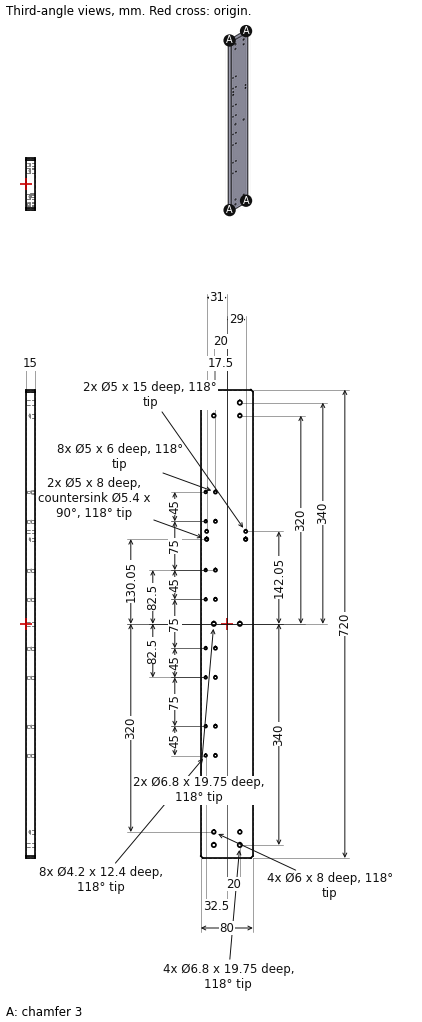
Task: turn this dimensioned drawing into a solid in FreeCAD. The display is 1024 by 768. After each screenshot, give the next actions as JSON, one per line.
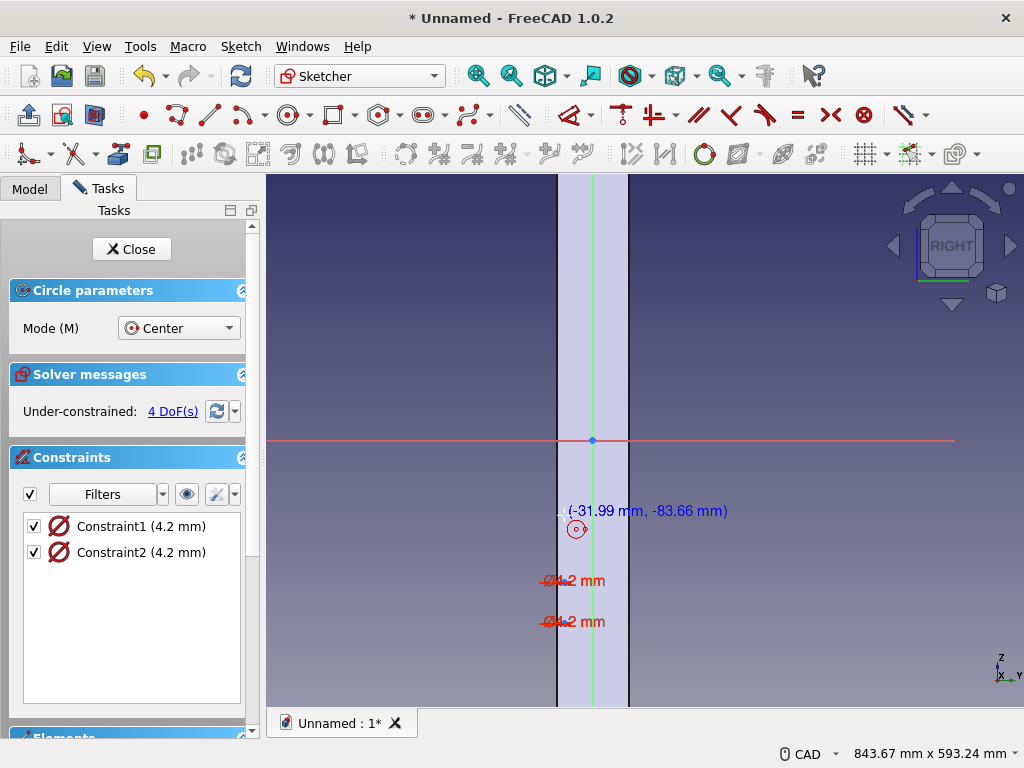
{"action": "left_click", "coordinate": [564, 515]}
{"action": "mouse_move", "coordinate": [565, 514]}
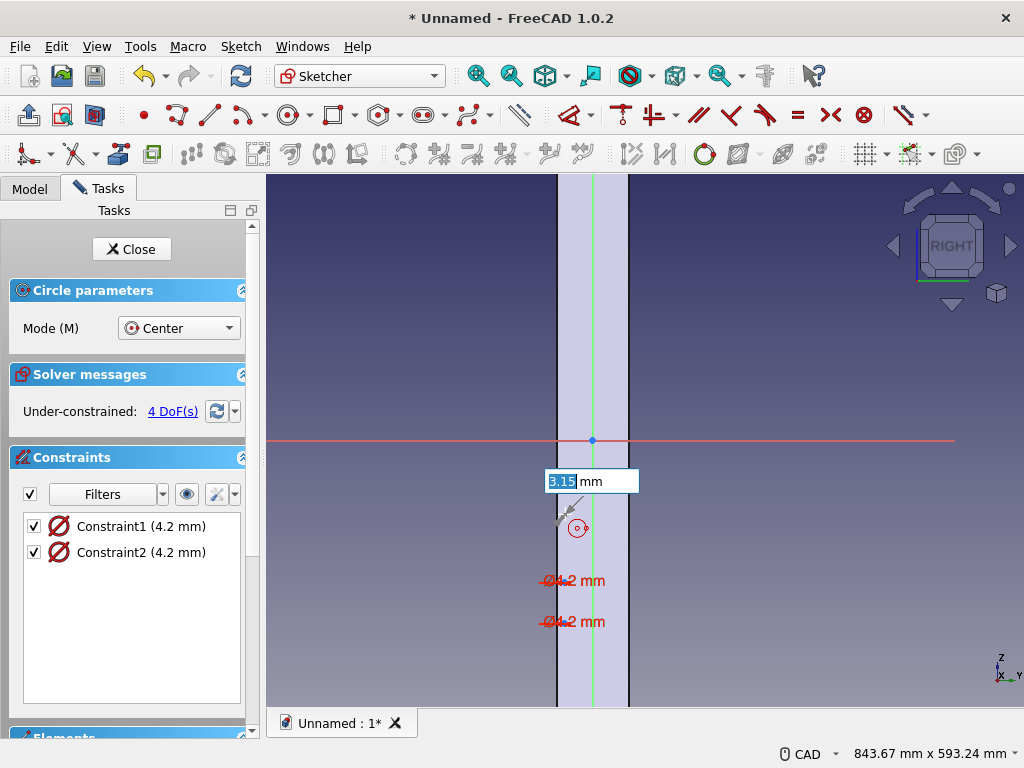
{"action": "type", "text": "4.2"}
{"action": "key", "text": "Return"}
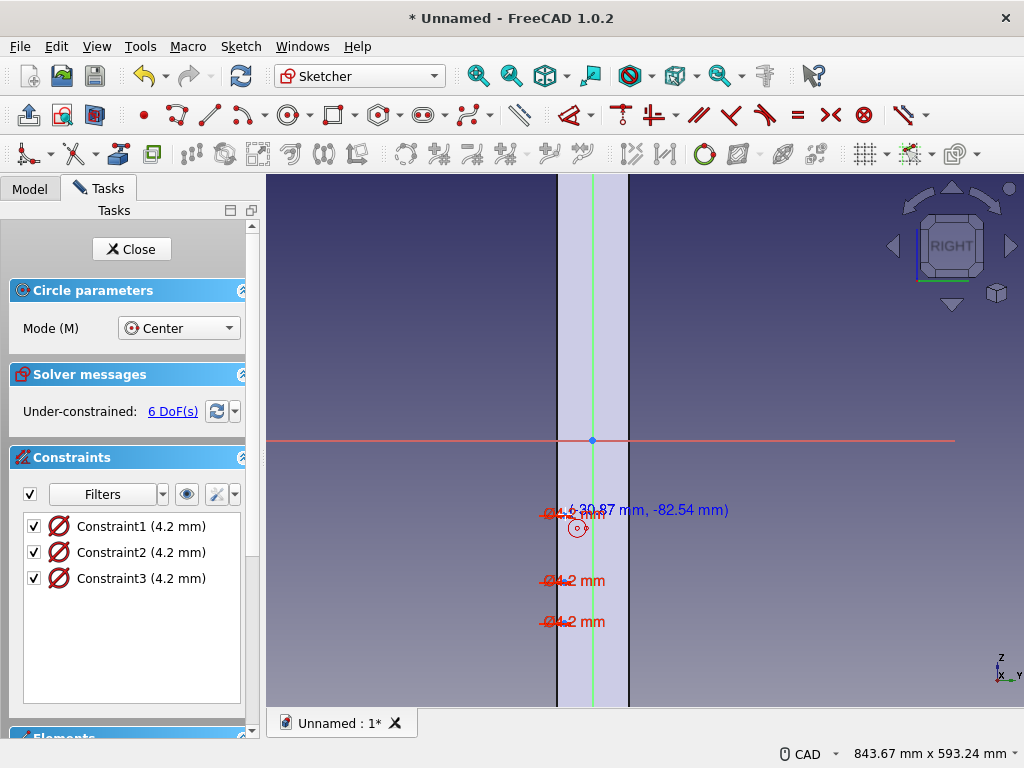
{"action": "scroll", "coordinate": [564, 475], "scroll_direction": "up", "scroll_amount": 13}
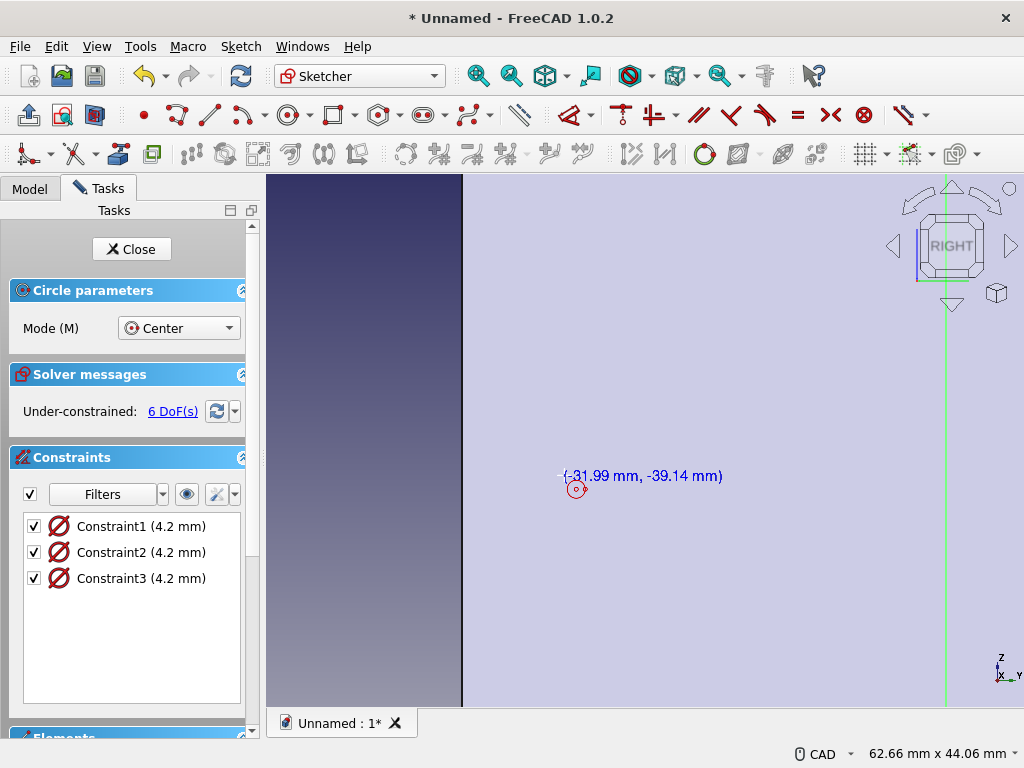
{"action": "scroll", "coordinate": [564, 475], "scroll_direction": "down", "scroll_amount": 13}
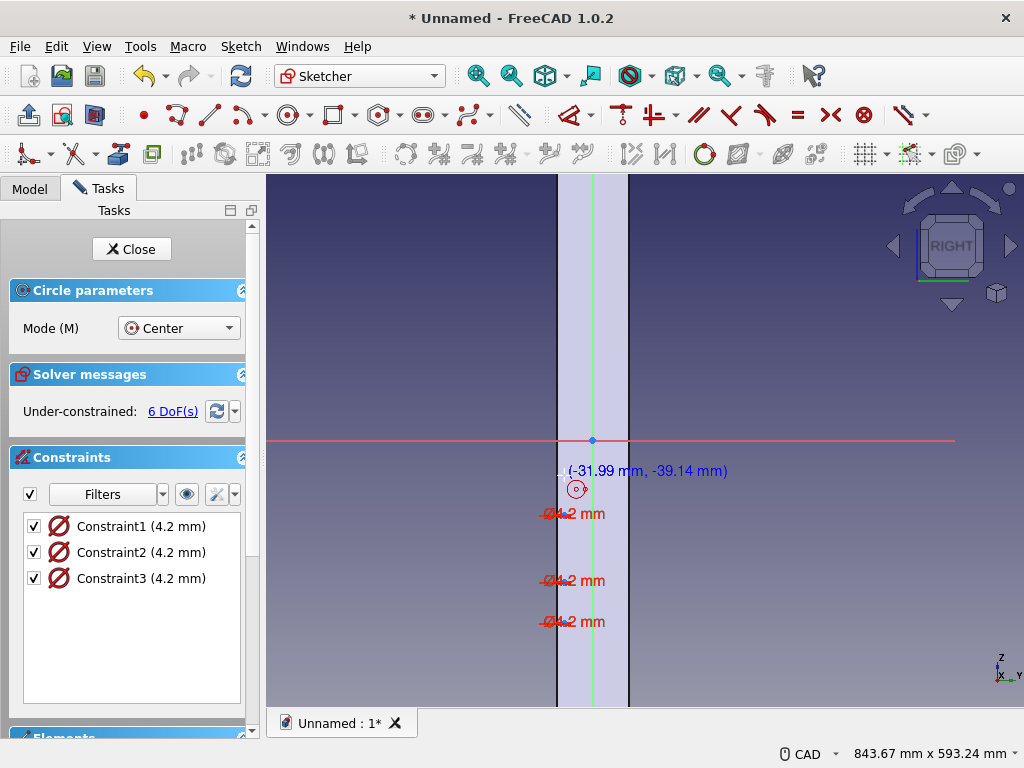
{"action": "left_click", "coordinate": [564, 475]}
{"action": "mouse_move", "coordinate": [565, 473]}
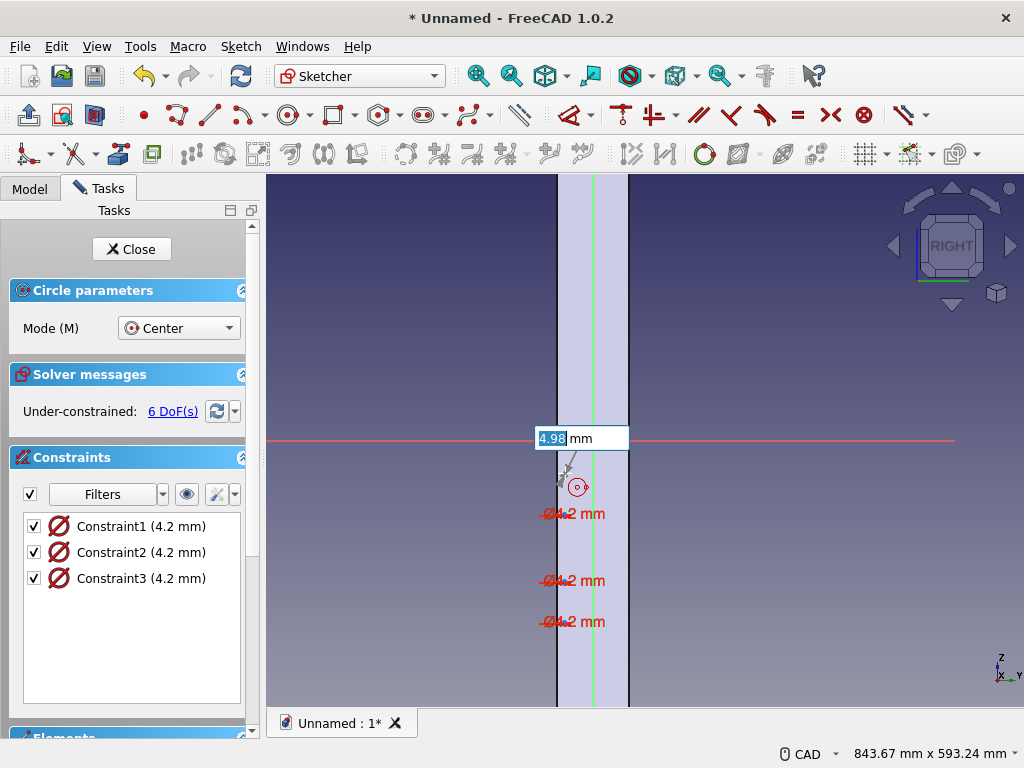
{"action": "type", "text": "4.2"}
{"action": "key", "text": "Return"}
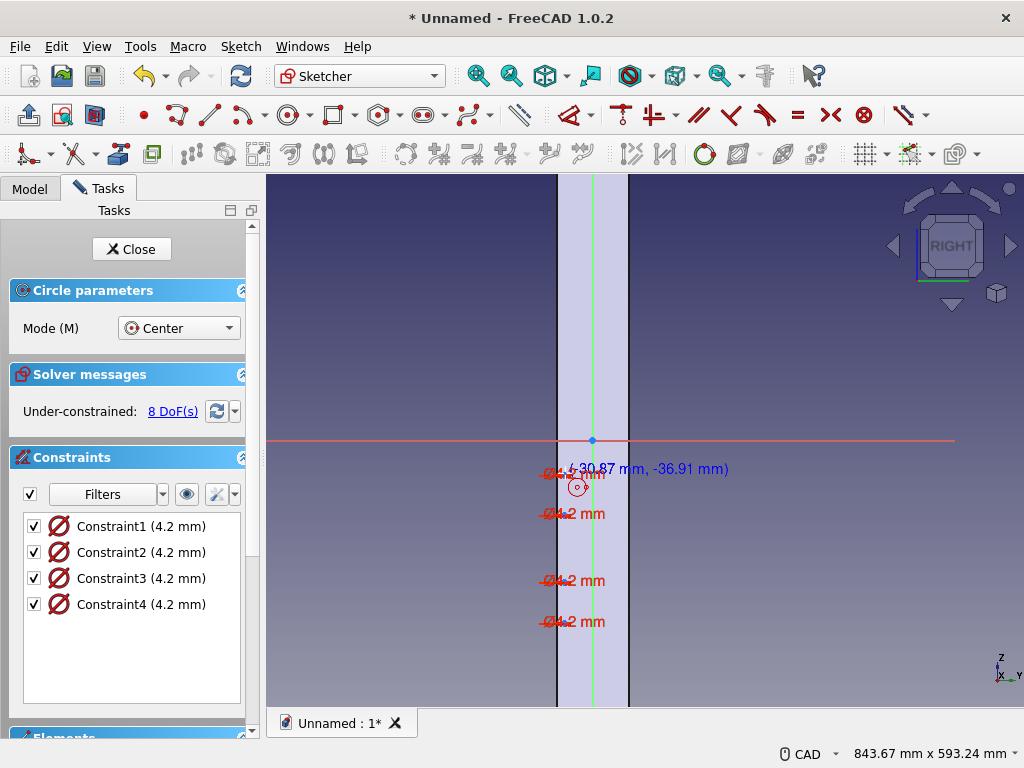
{"action": "scroll", "coordinate": [564, 407], "scroll_direction": "up", "scroll_amount": 13}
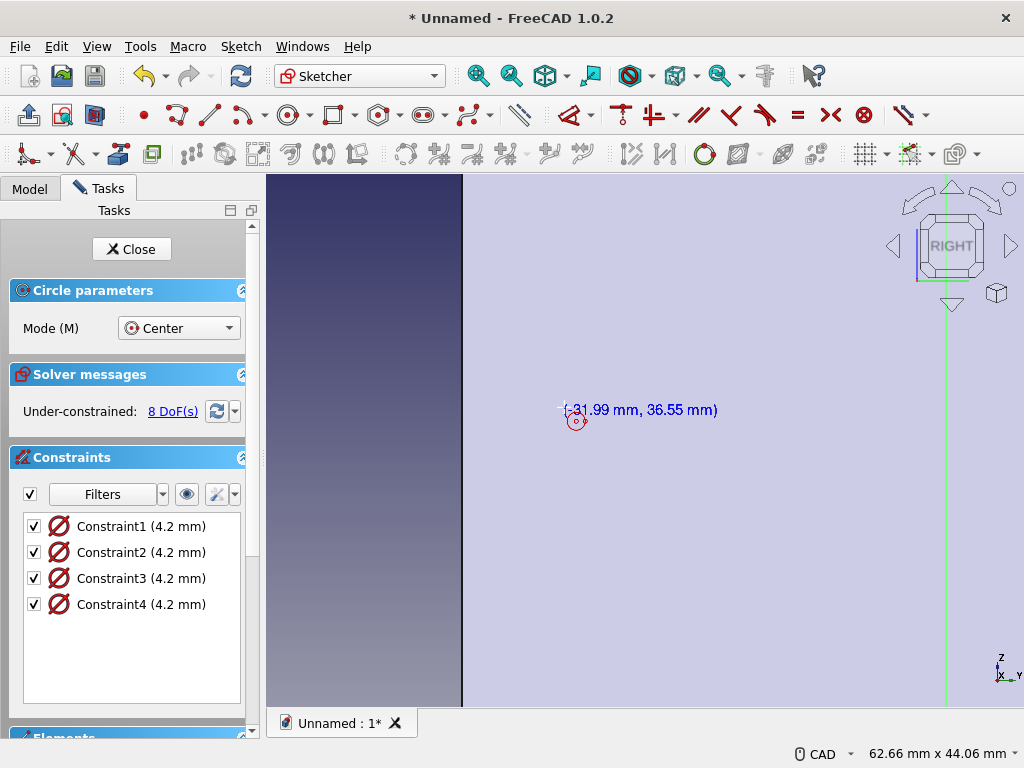
{"action": "scroll", "coordinate": [564, 407], "scroll_direction": "down", "scroll_amount": 13}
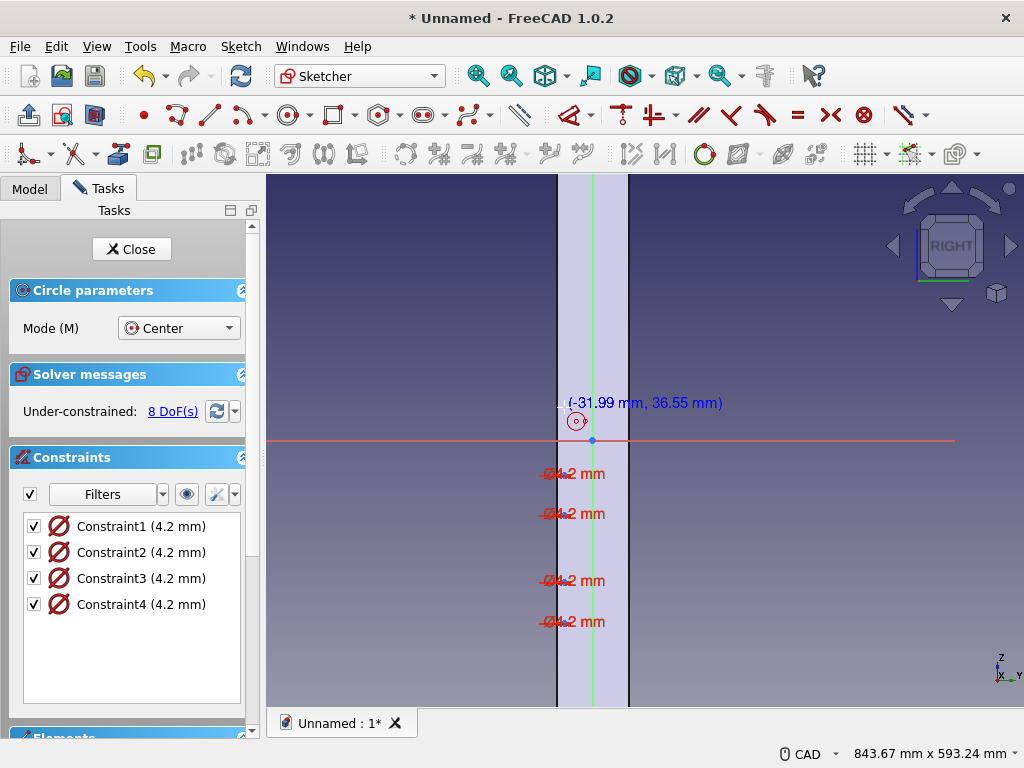
{"action": "left_click", "coordinate": [564, 407]}
{"action": "mouse_move", "coordinate": [565, 406]}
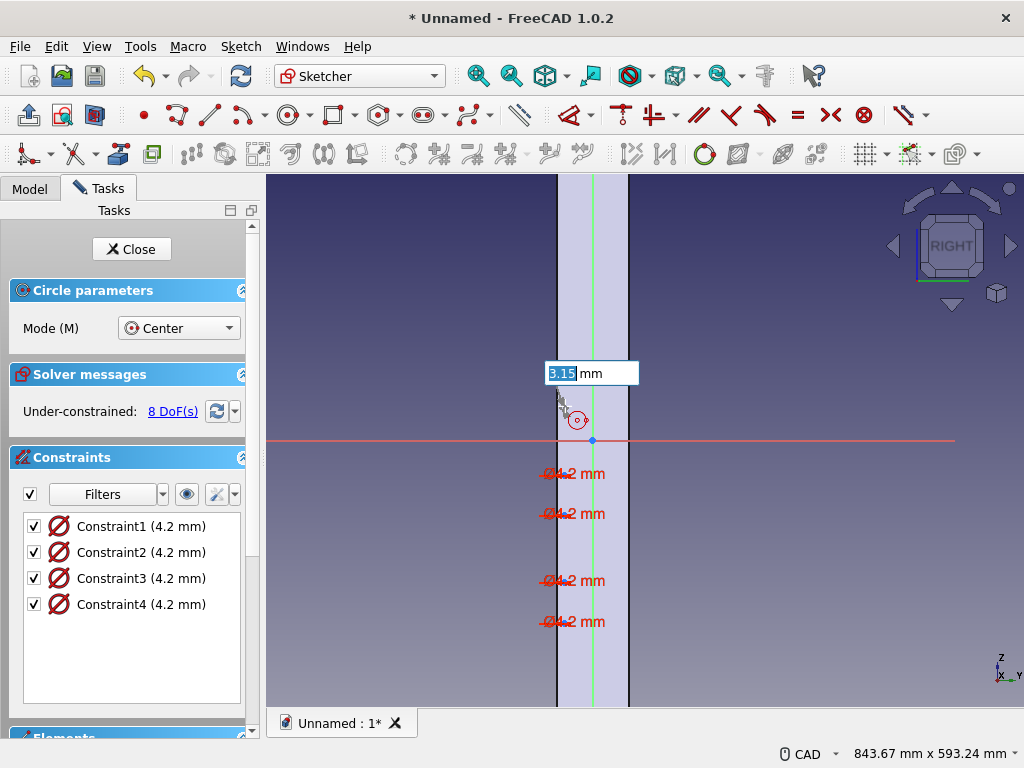
{"action": "type", "text": "4.2"}
{"action": "key", "text": "Return"}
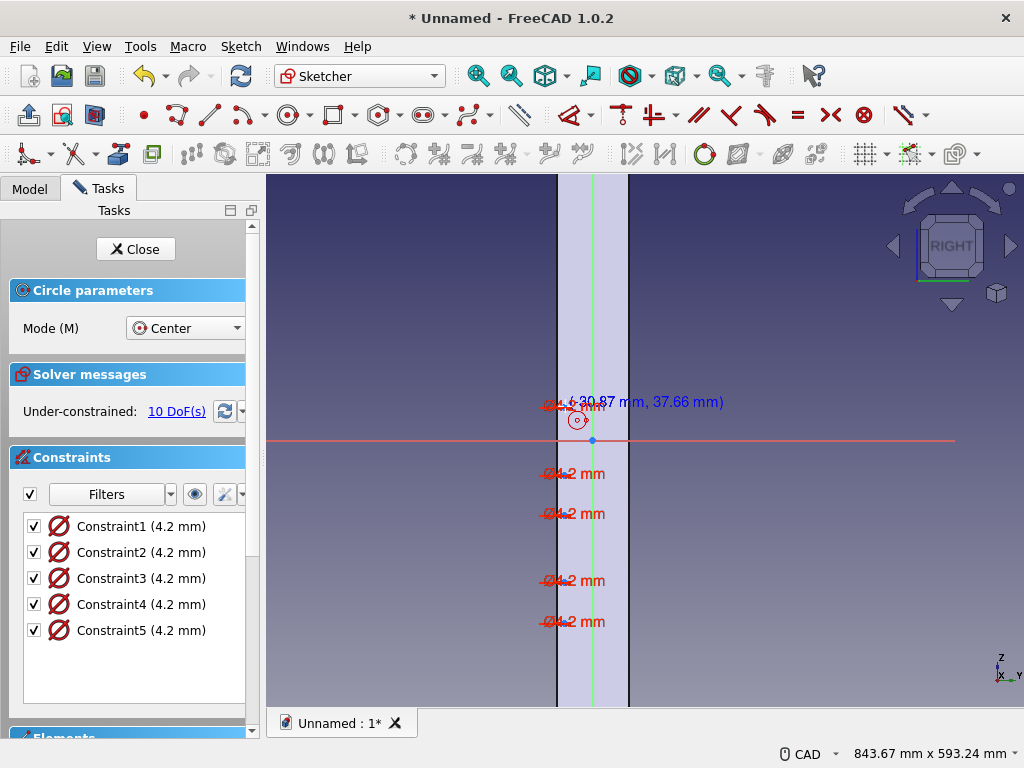
{"action": "scroll", "coordinate": [564, 367], "scroll_direction": "up", "scroll_amount": 13}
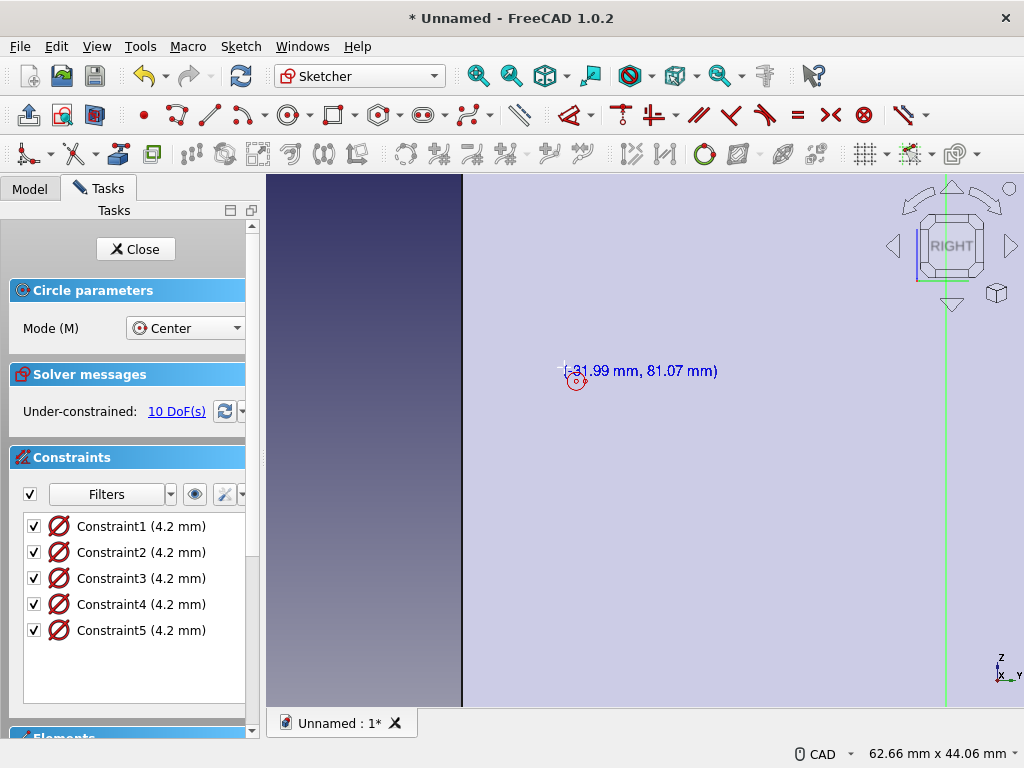
{"action": "scroll", "coordinate": [564, 367], "scroll_direction": "down", "scroll_amount": 13}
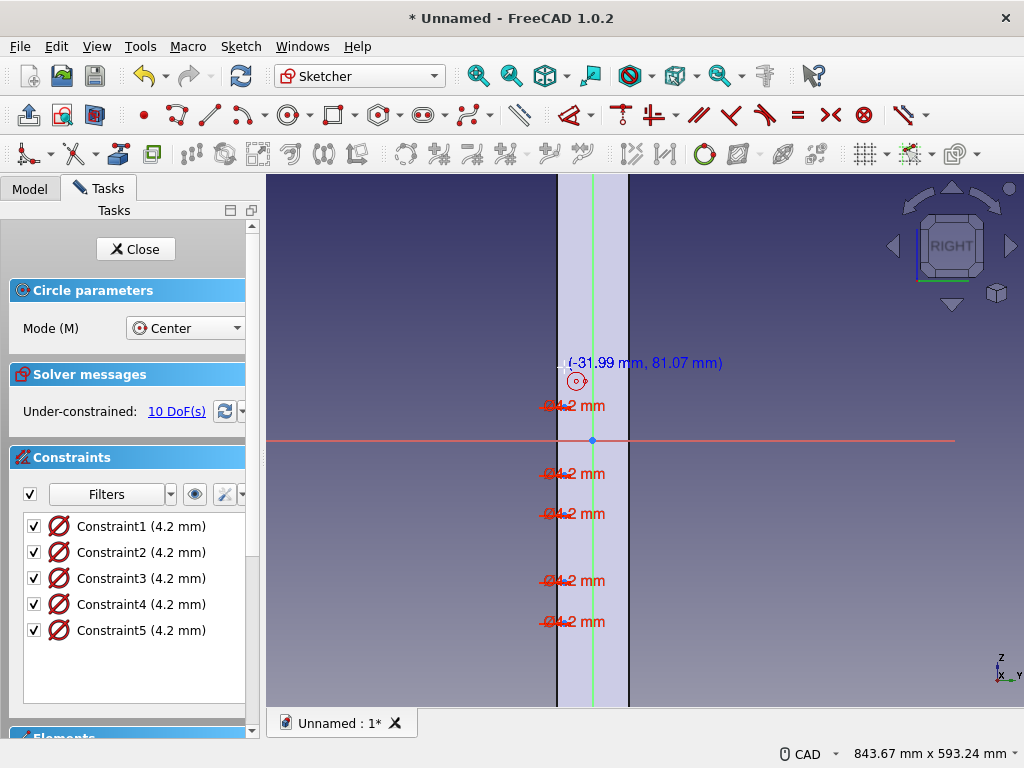
{"action": "left_click", "coordinate": [564, 367]}
{"action": "mouse_move", "coordinate": [565, 365]}